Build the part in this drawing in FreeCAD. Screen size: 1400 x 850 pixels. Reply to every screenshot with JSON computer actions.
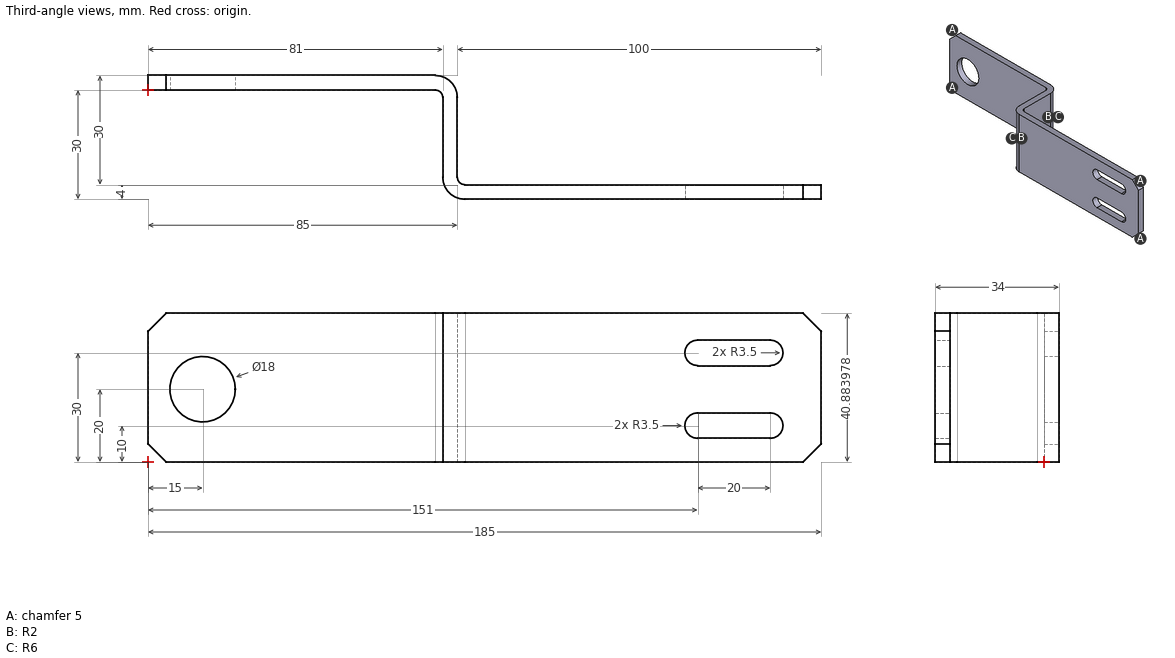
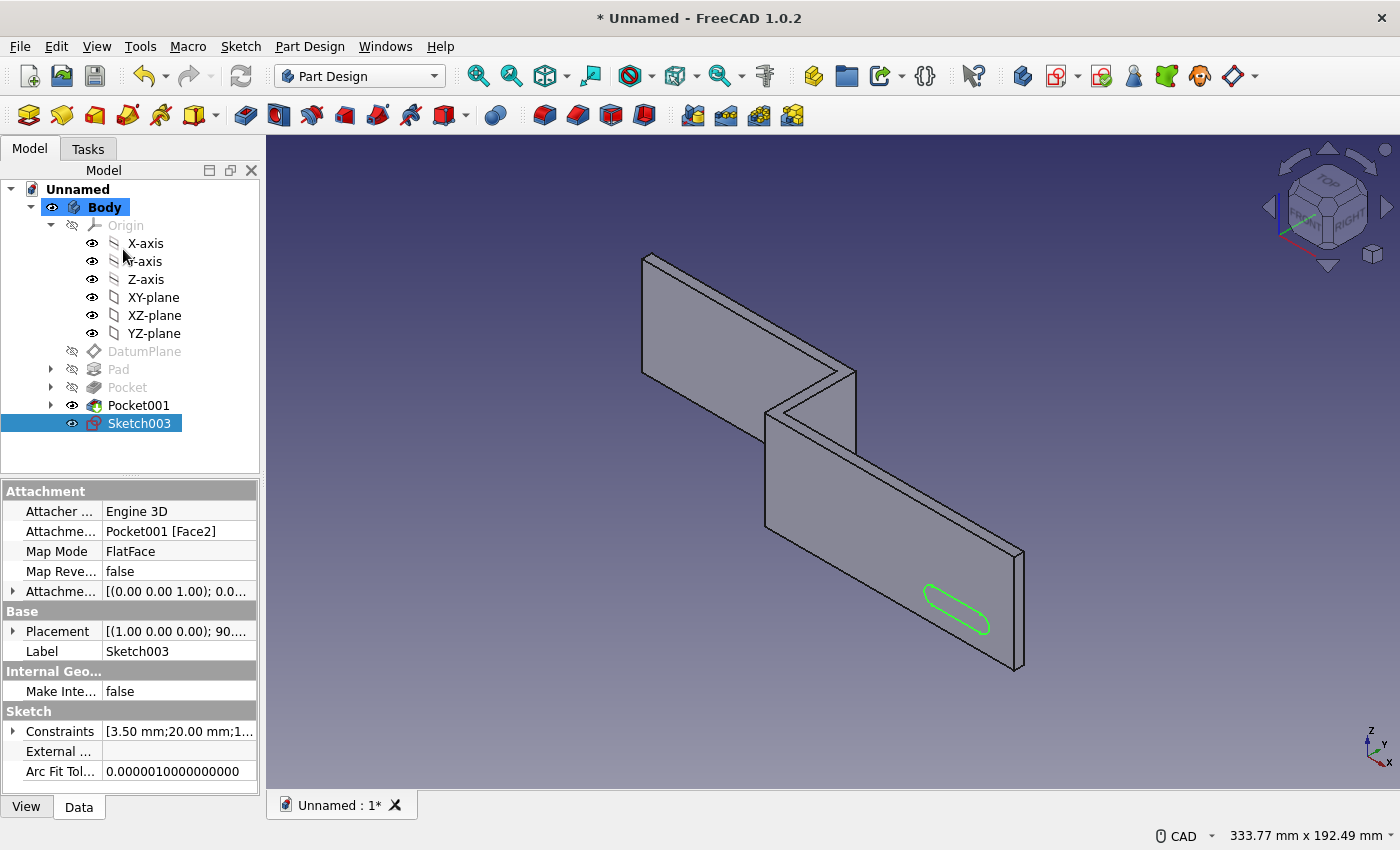
{"action": "left_click", "coordinate": [246, 116]}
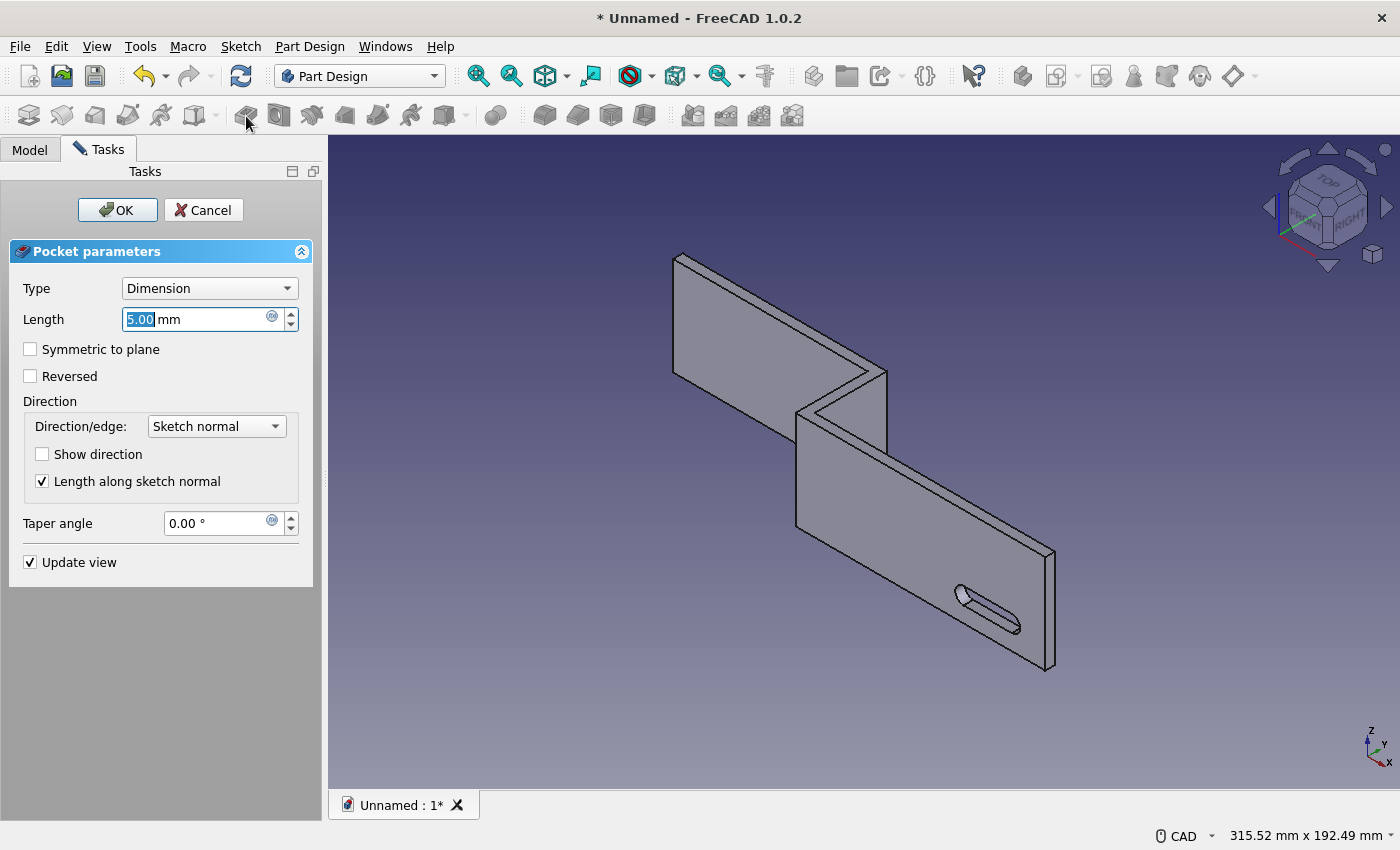
{"action": "left_click", "coordinate": [210, 288]}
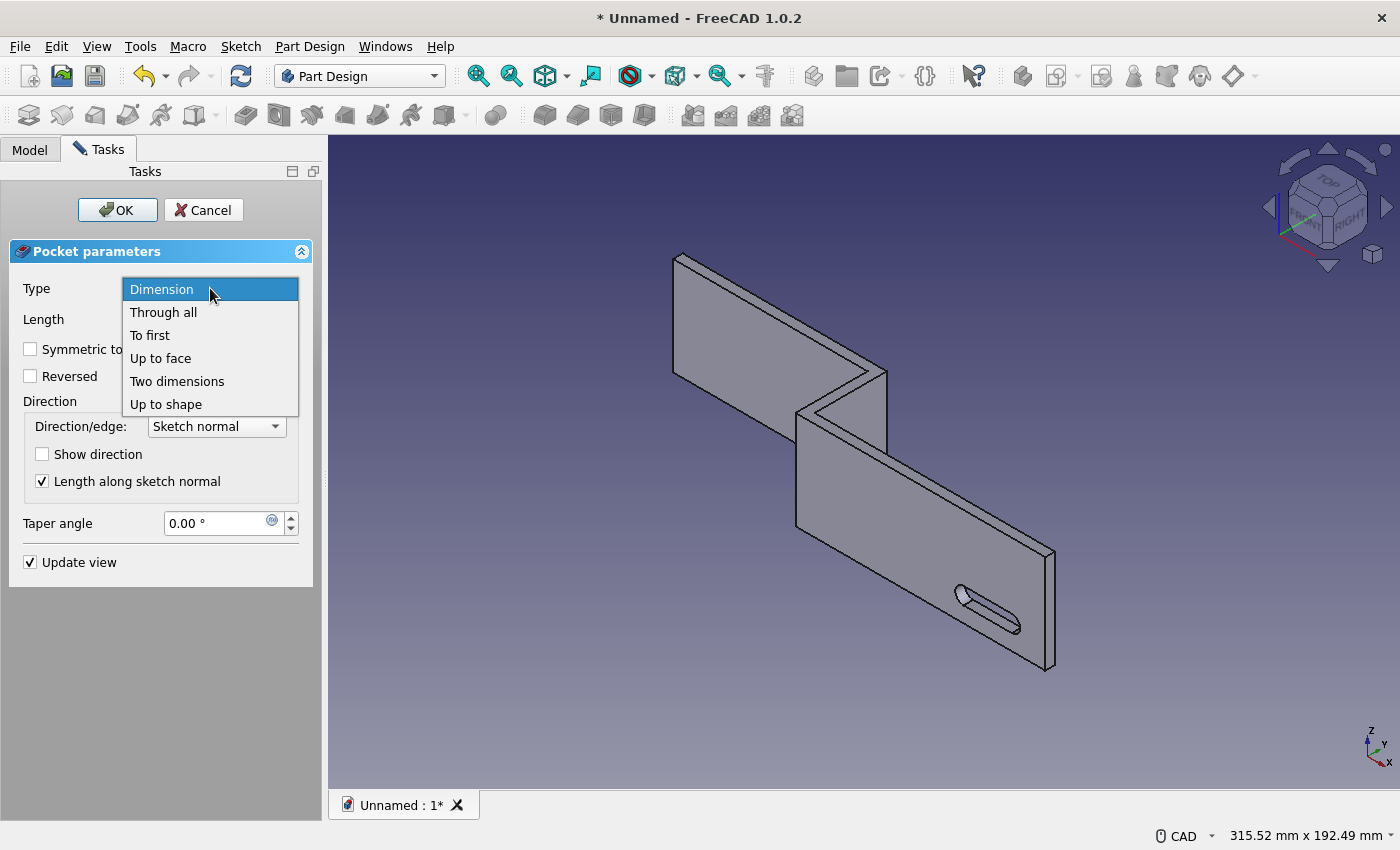
{"action": "left_click", "coordinate": [208, 312]}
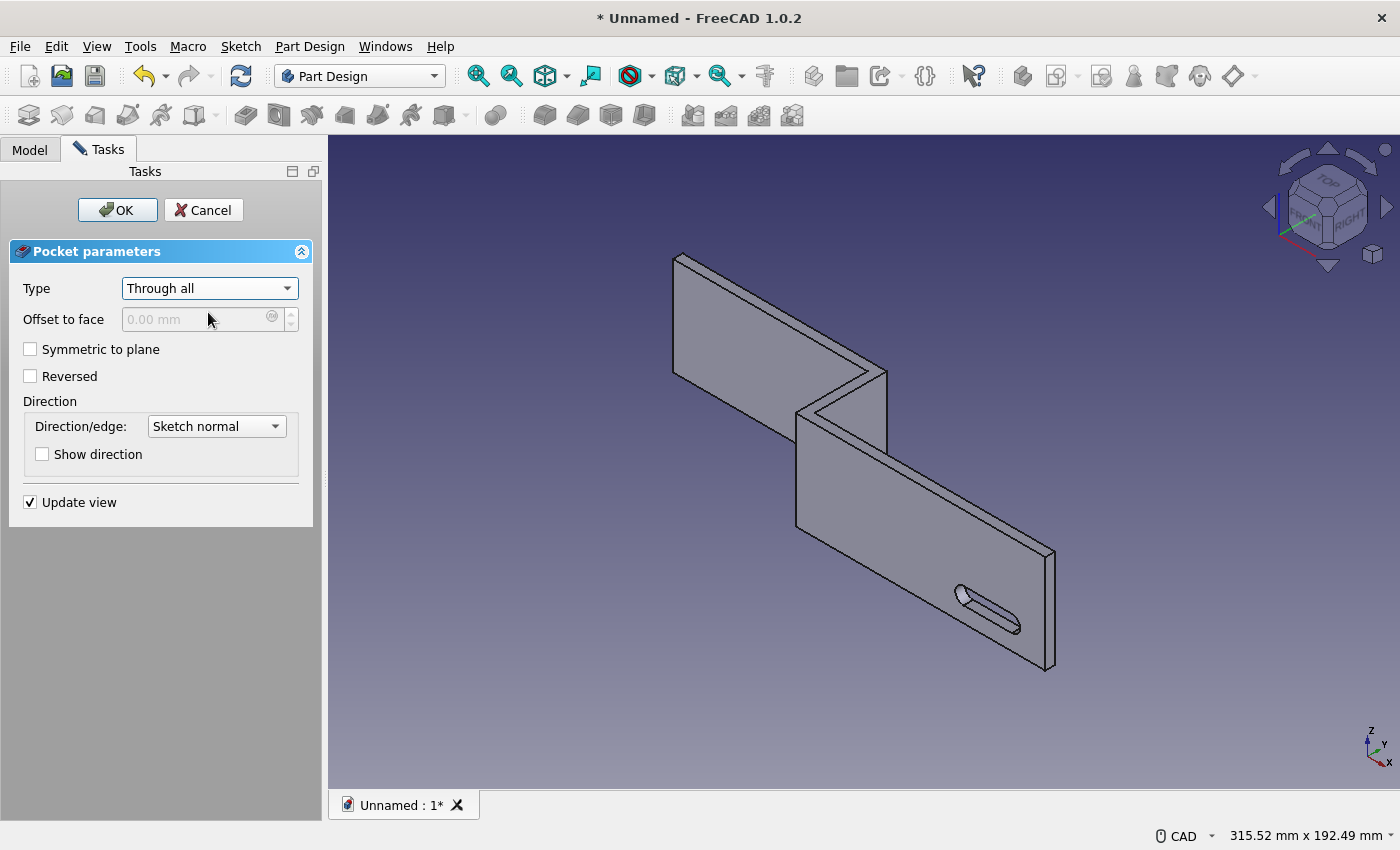
{"action": "left_click", "coordinate": [118, 210]}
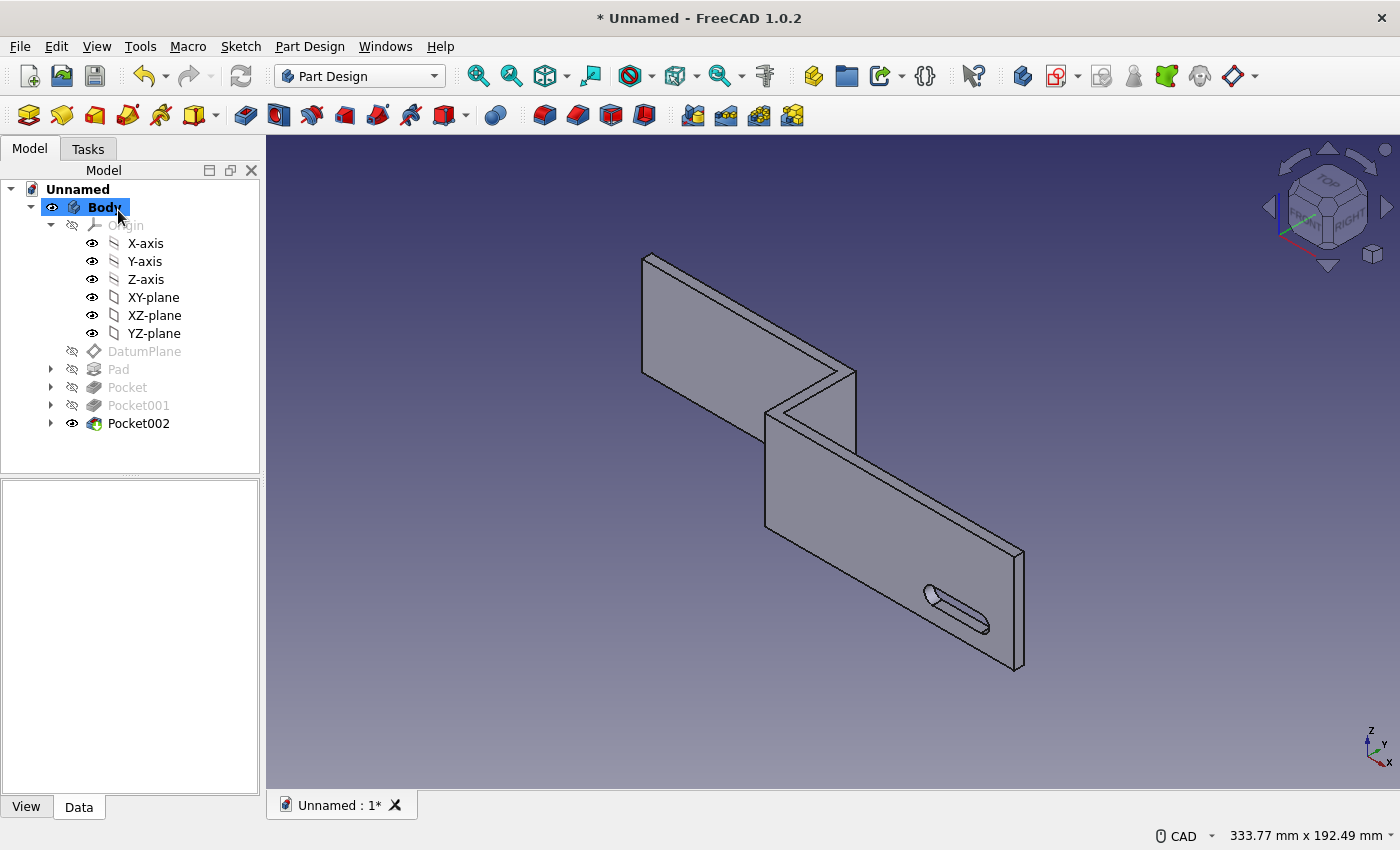
{"action": "key", "text": "4"}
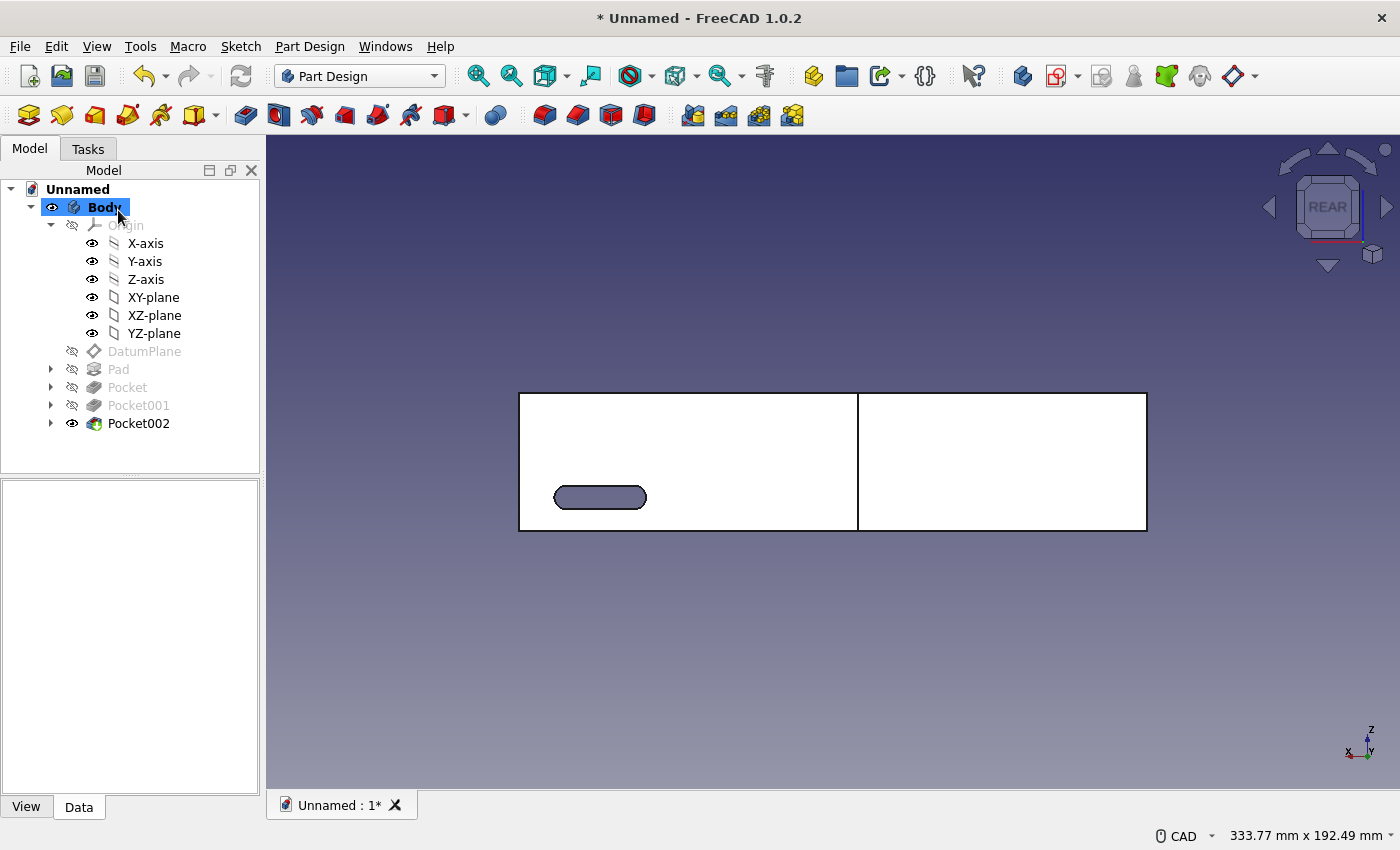
{"action": "left_click", "coordinate": [737, 461]}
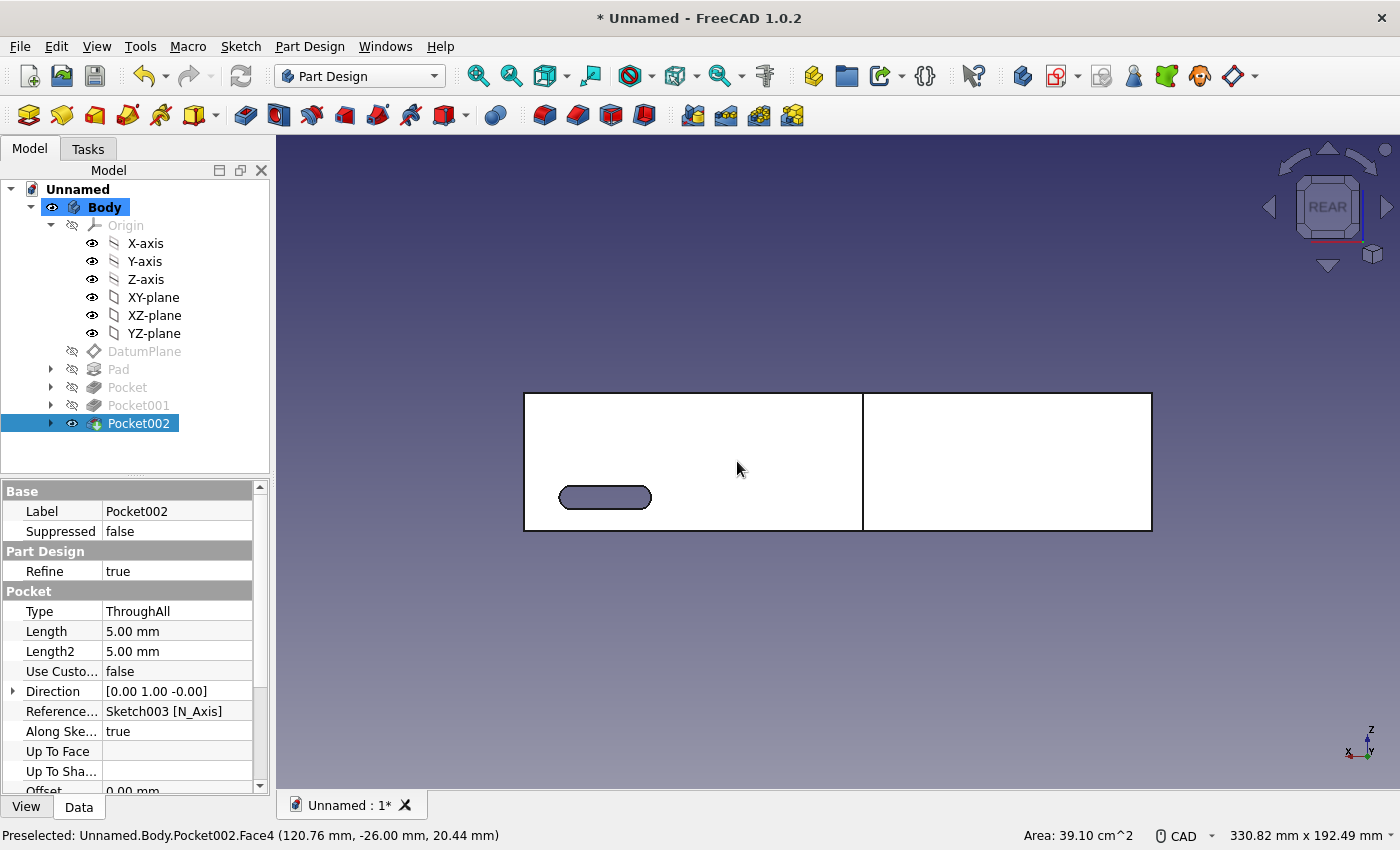
{"action": "left_click", "coordinate": [1056, 76]}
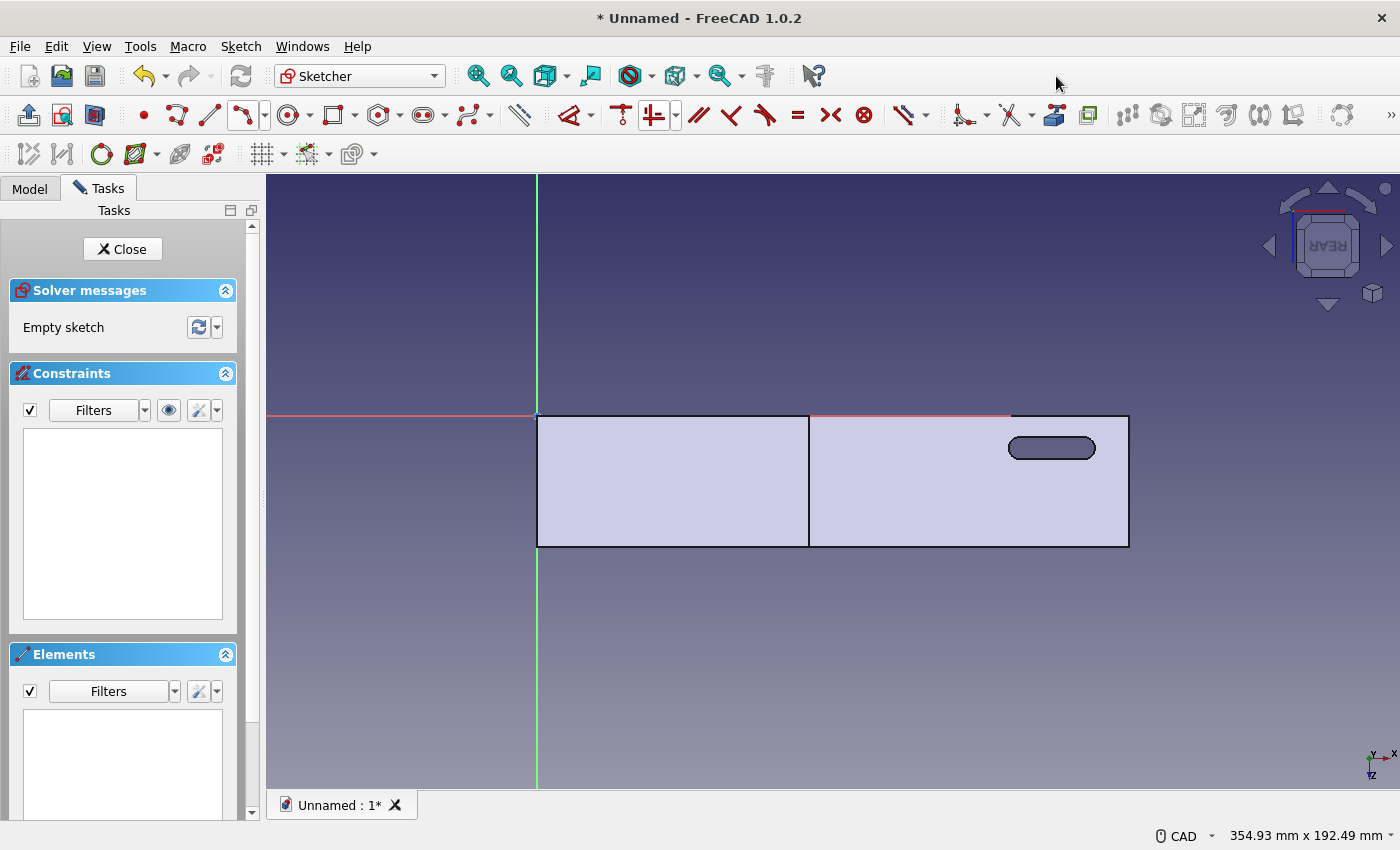
{"action": "left_click", "coordinate": [95, 116]}